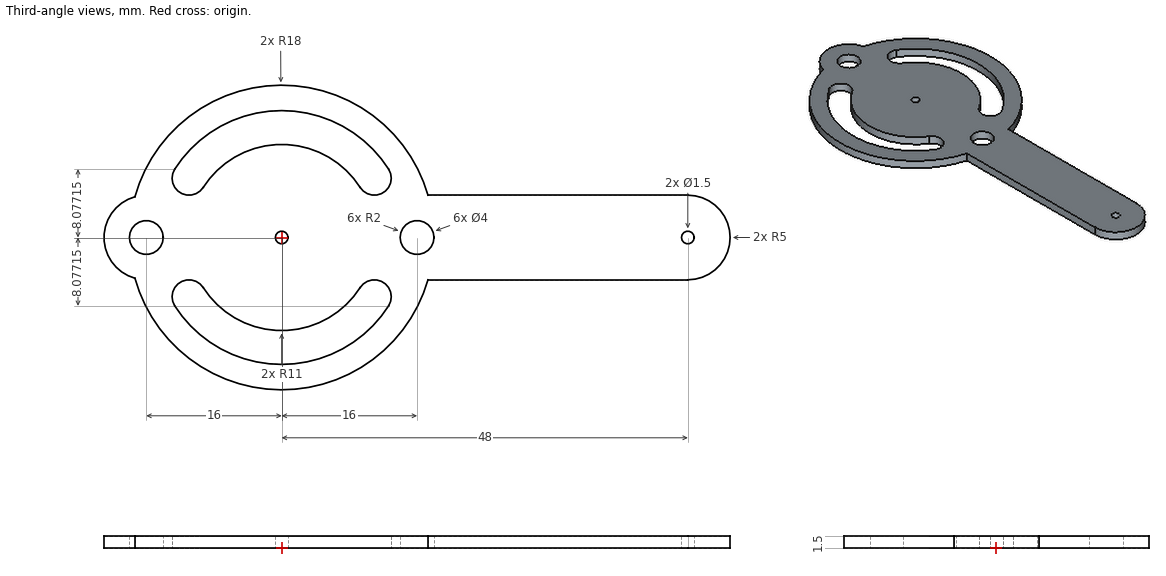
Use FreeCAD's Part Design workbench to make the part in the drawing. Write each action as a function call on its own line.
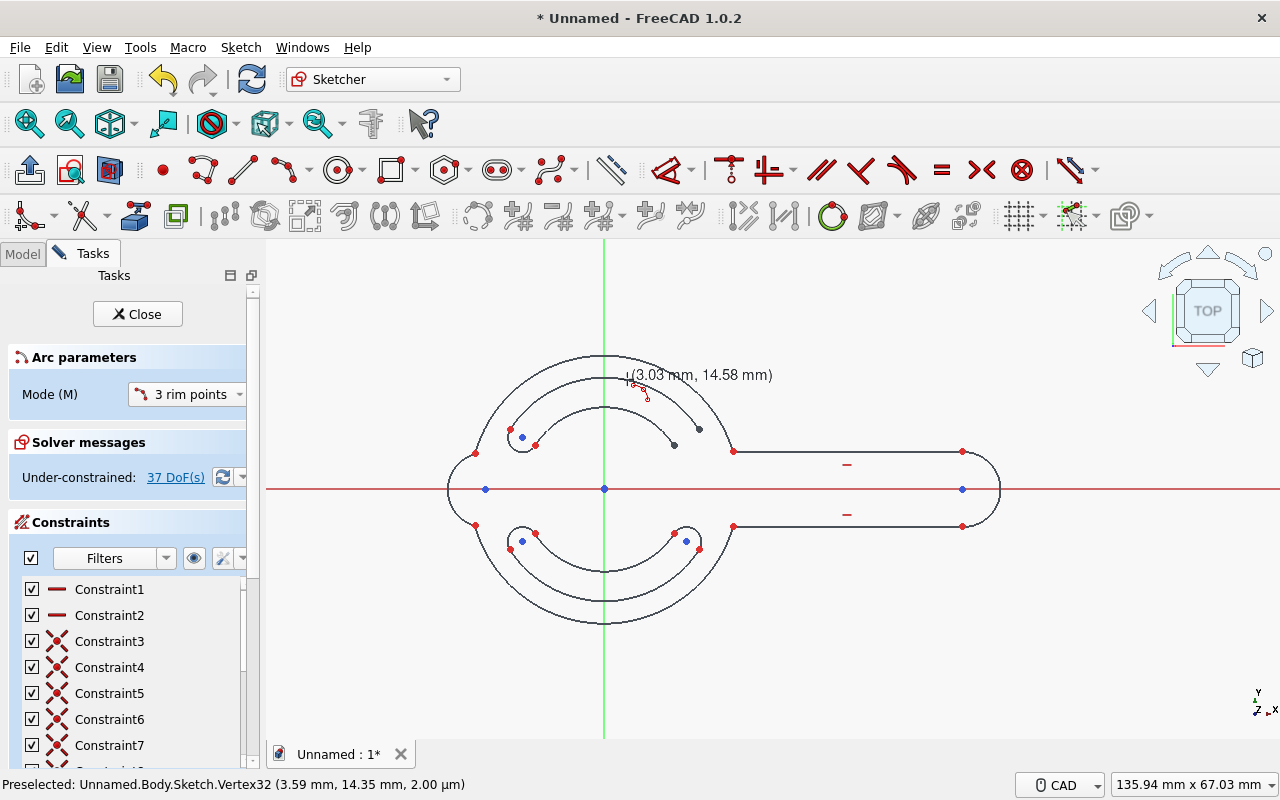
click(699, 430)
click(674, 446)
click(694, 449)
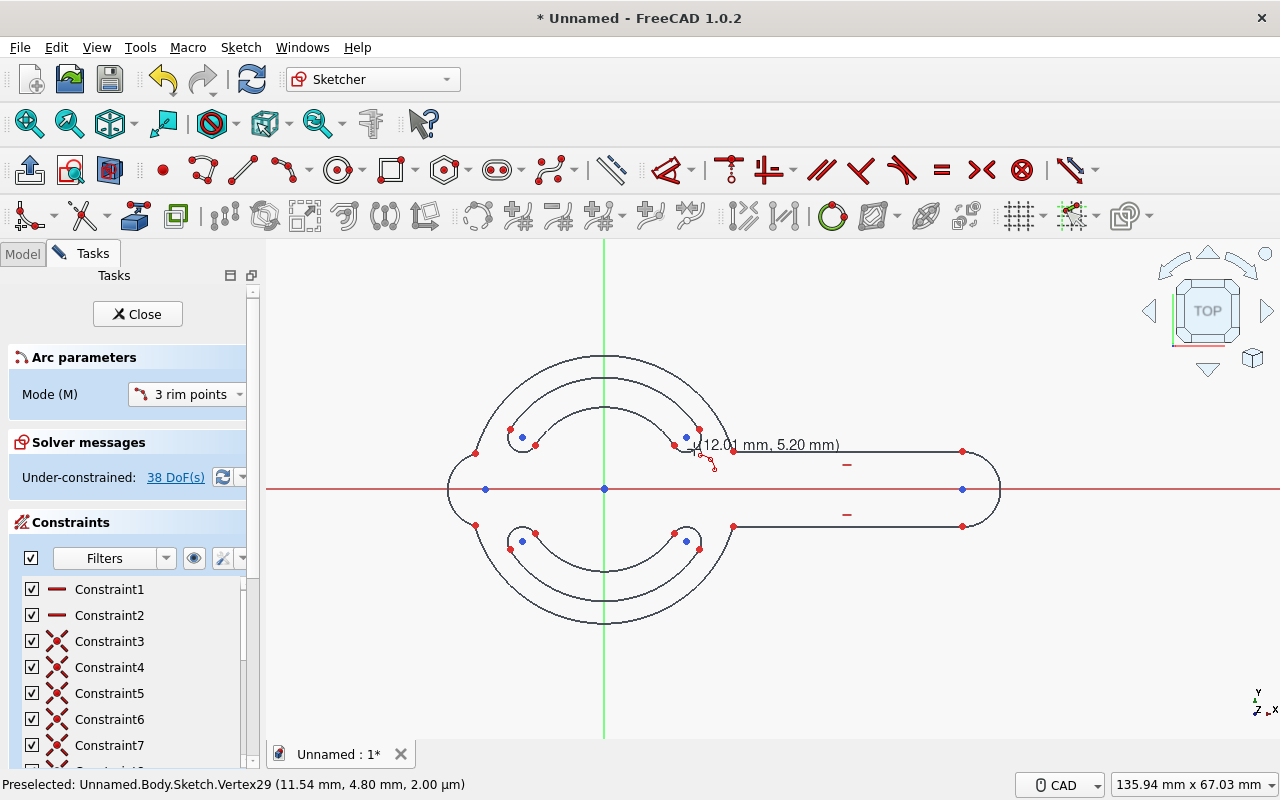
click(338, 170)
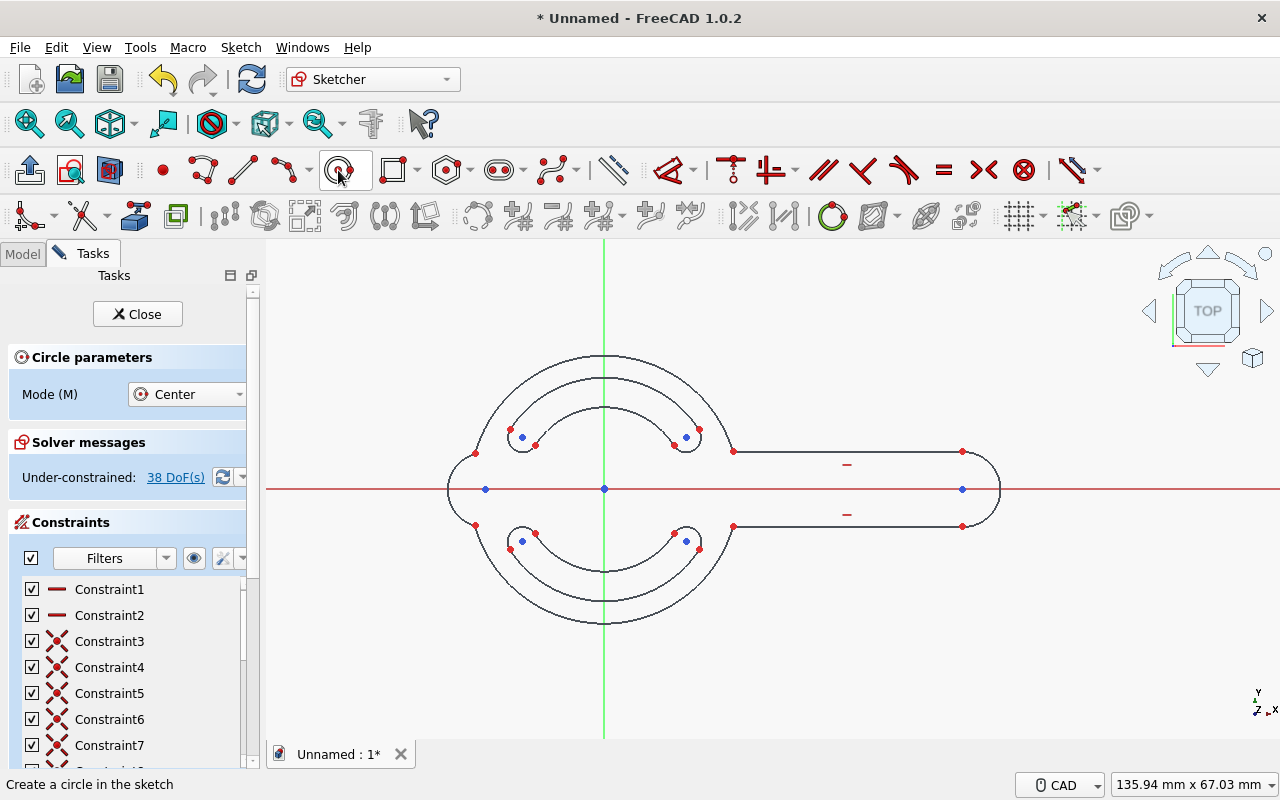
scroll(962, 489, up, 7)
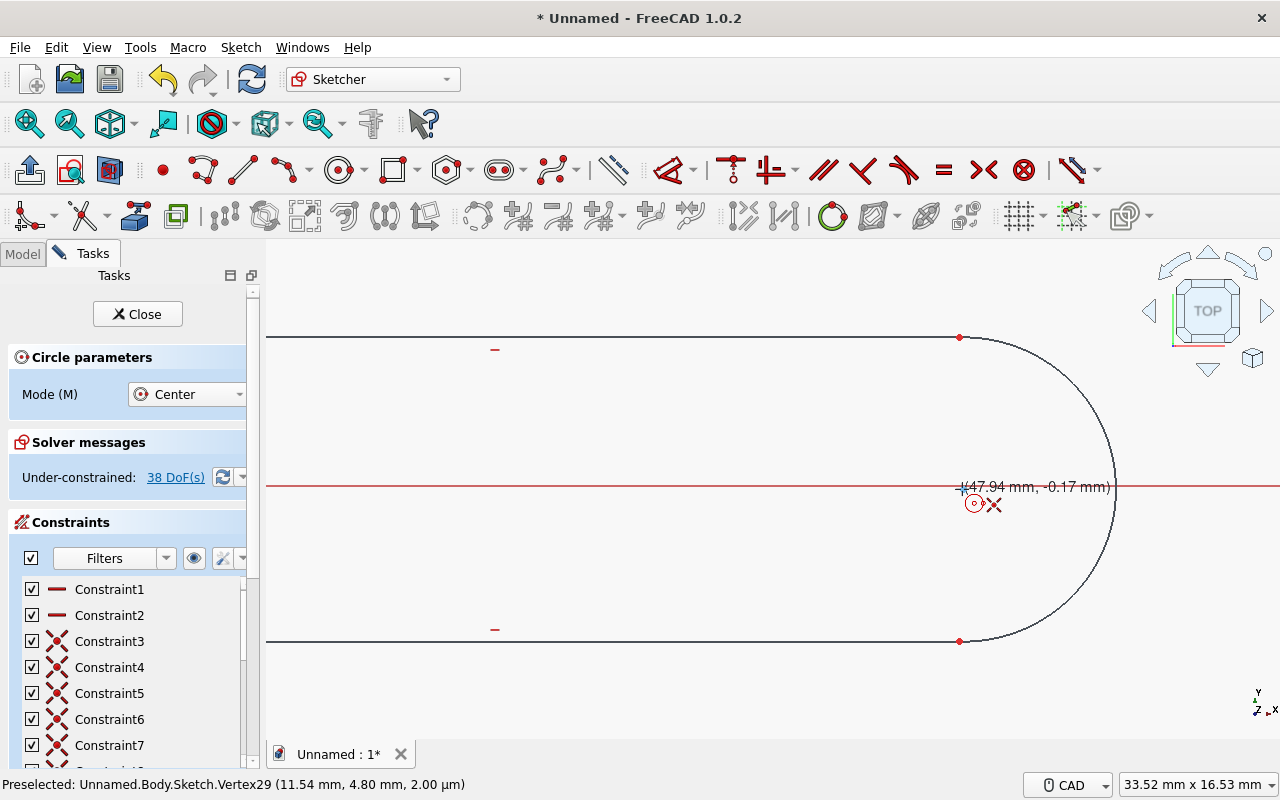
scroll(937, 490, down, 7)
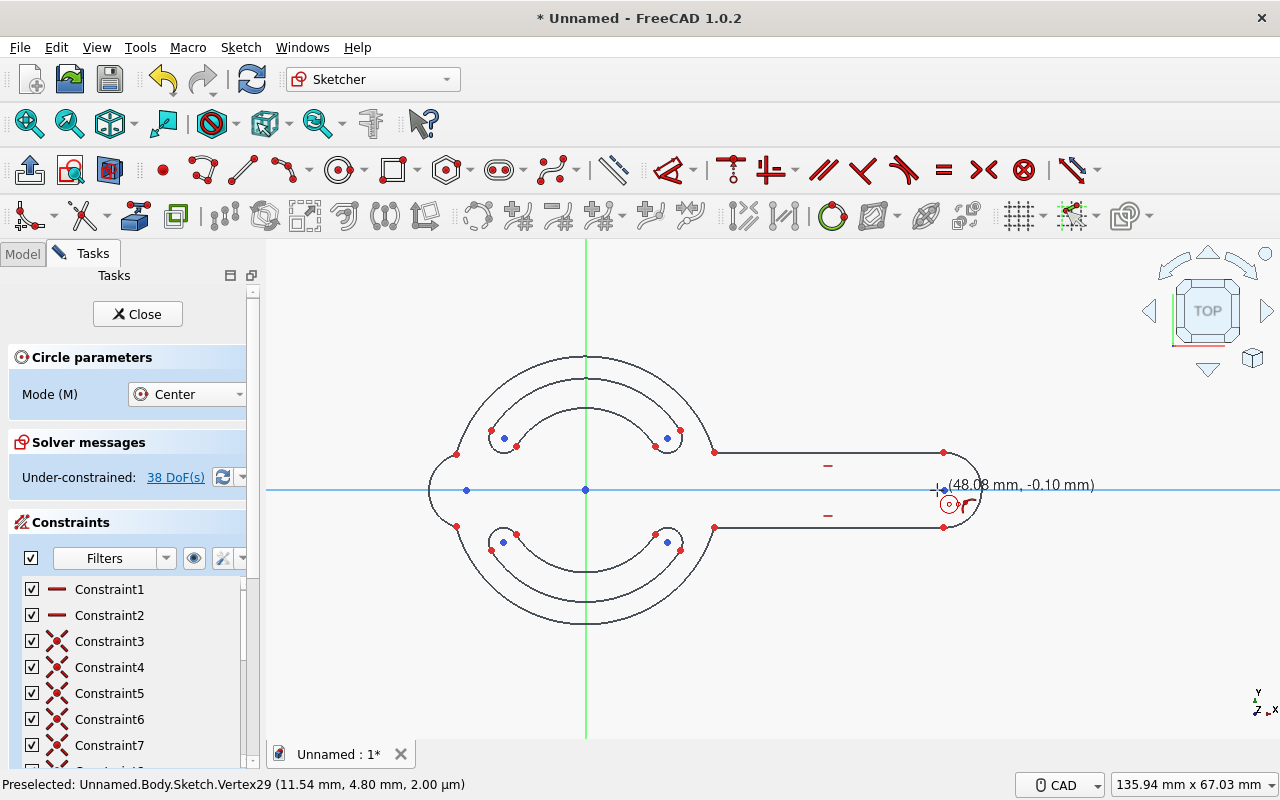
click(944, 490)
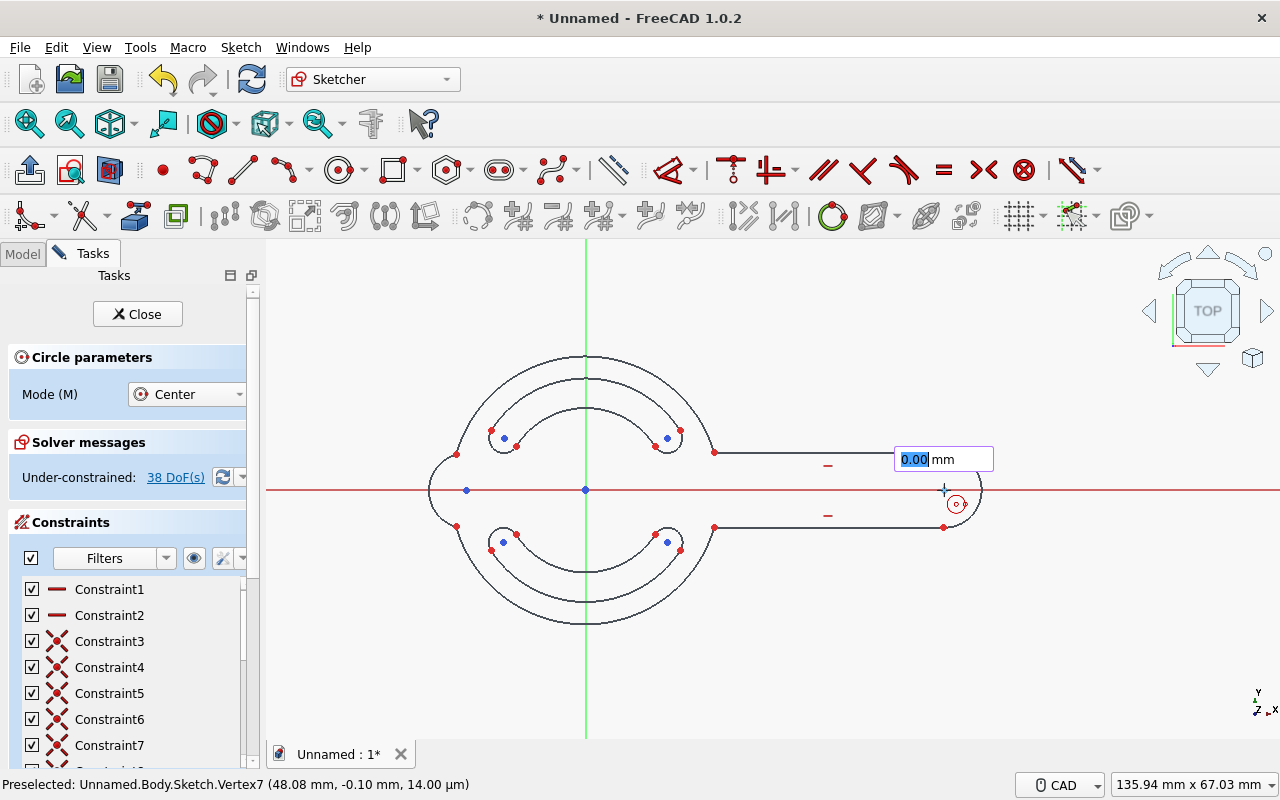
scroll(942, 495, up, 6)
move(939, 493)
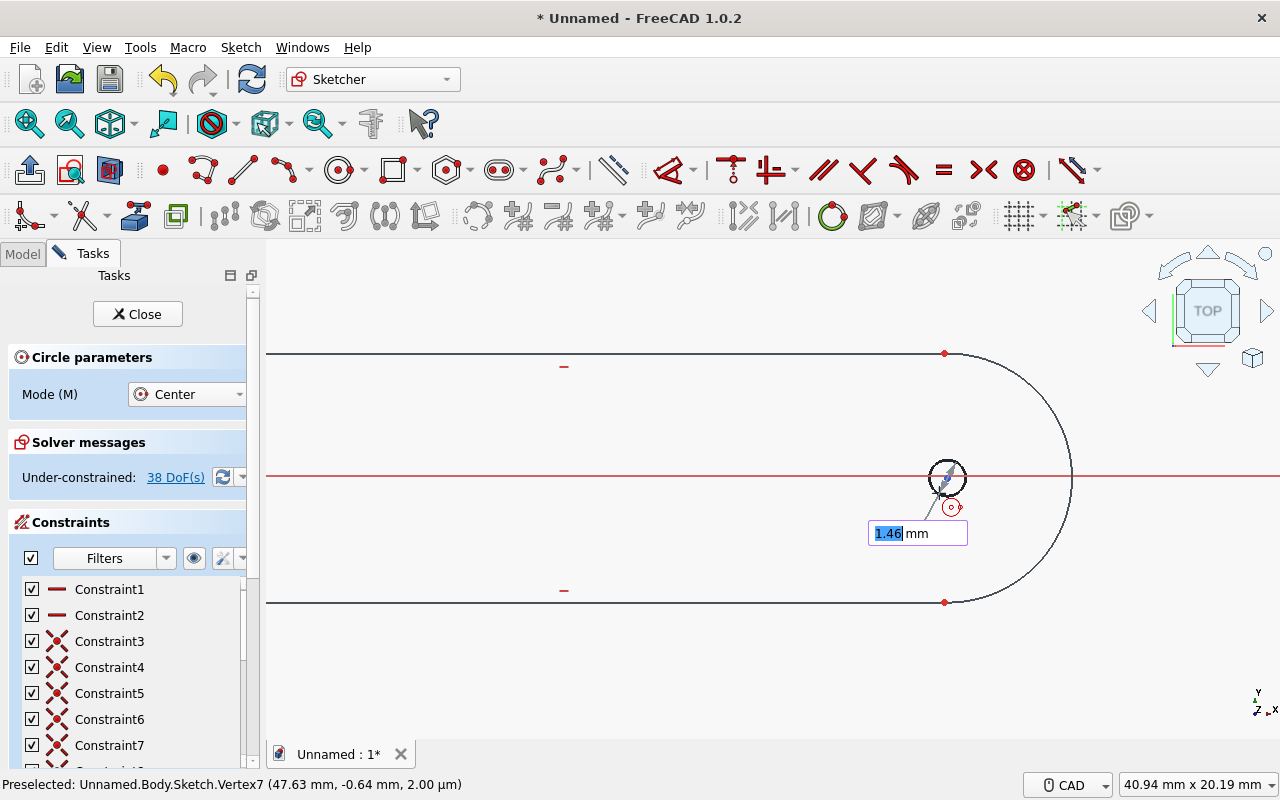
text(1.5)
key(Return)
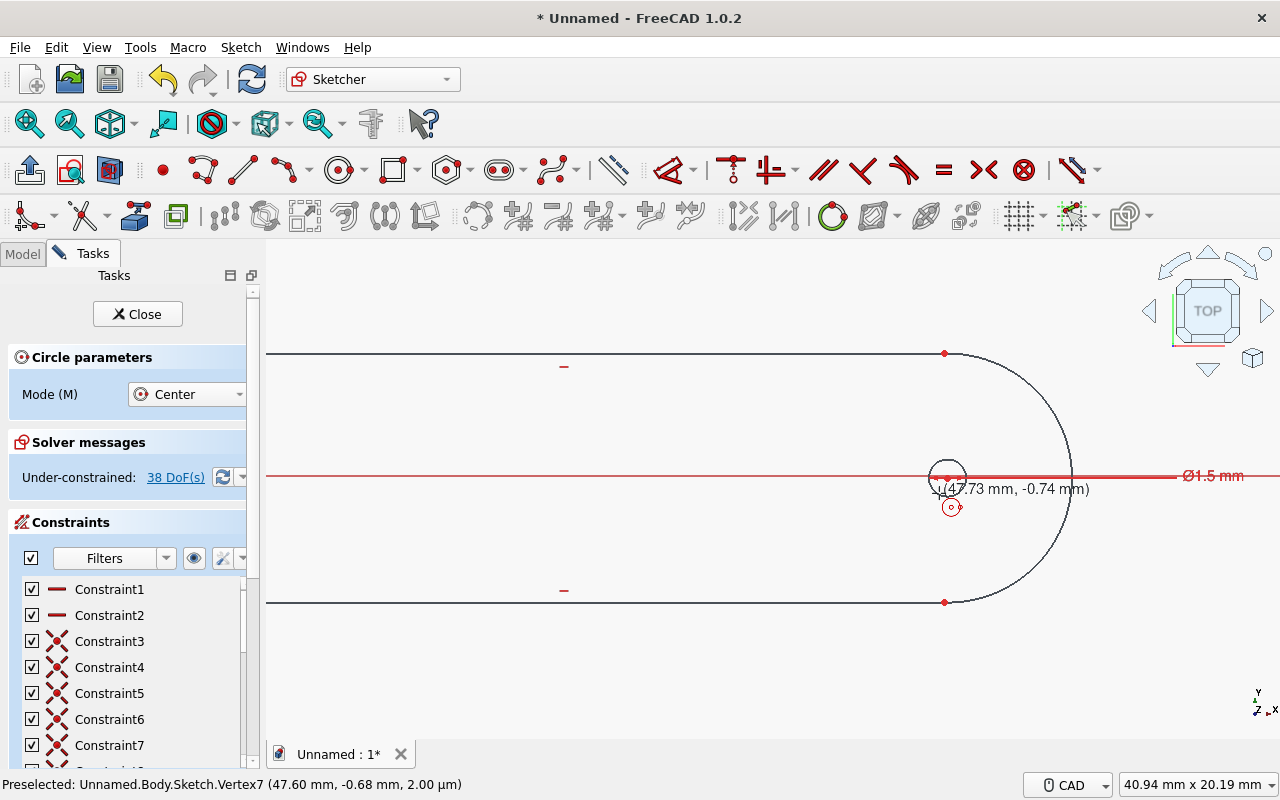
scroll(942, 495, down, 6)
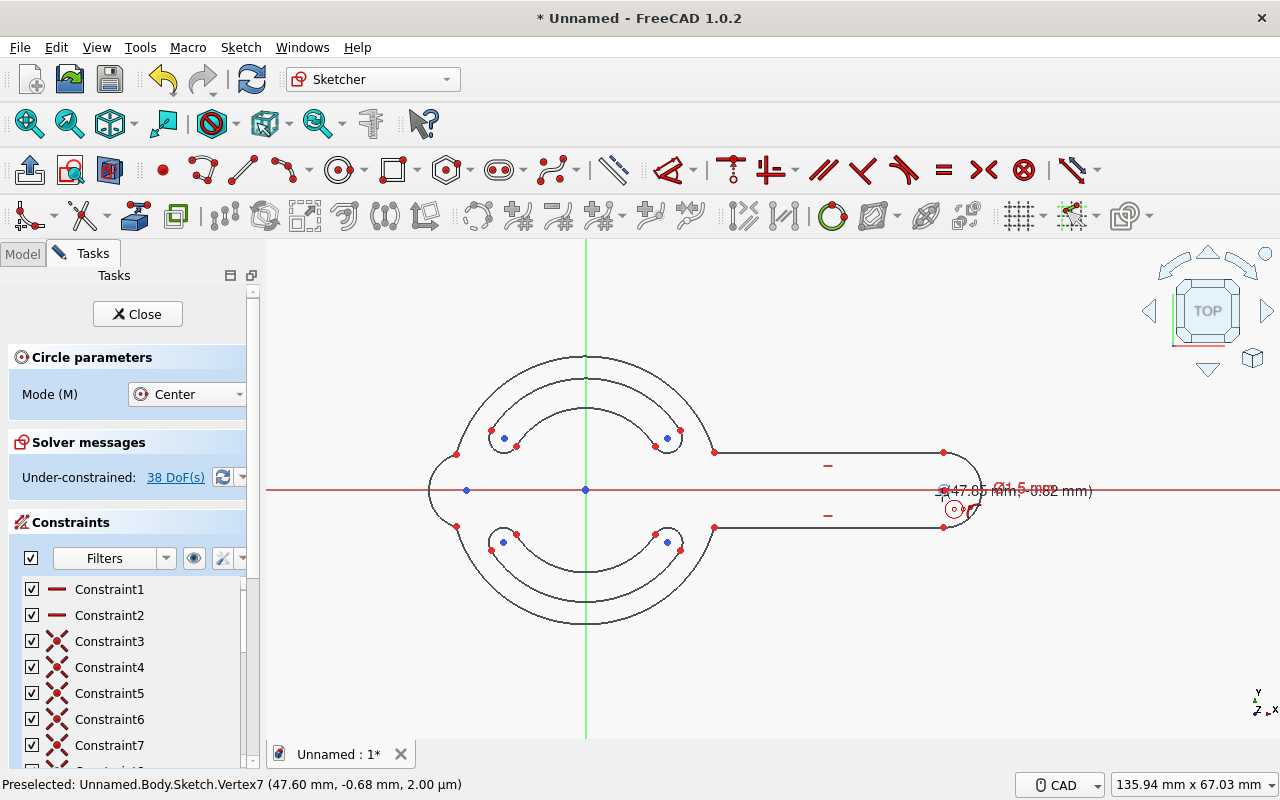
scroll(705, 490, up, 3)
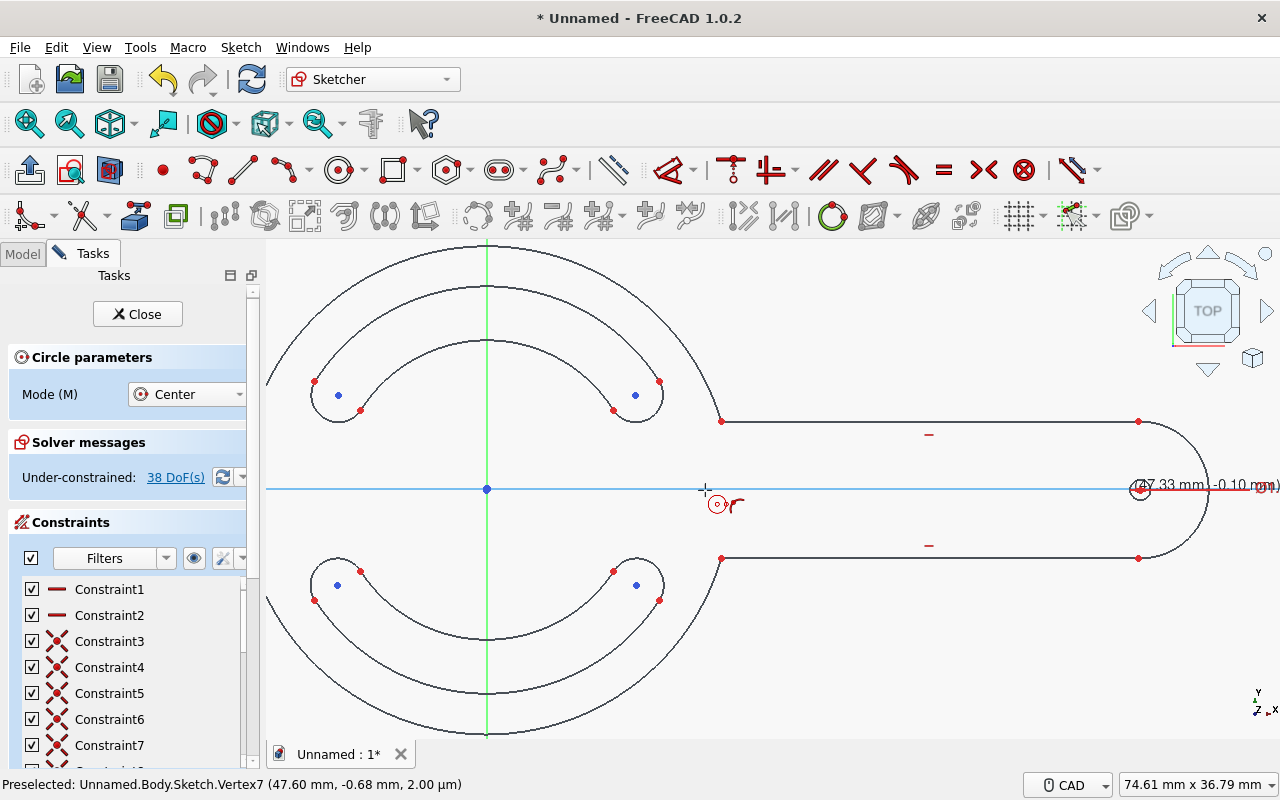
click(704, 489)
move(724, 469)